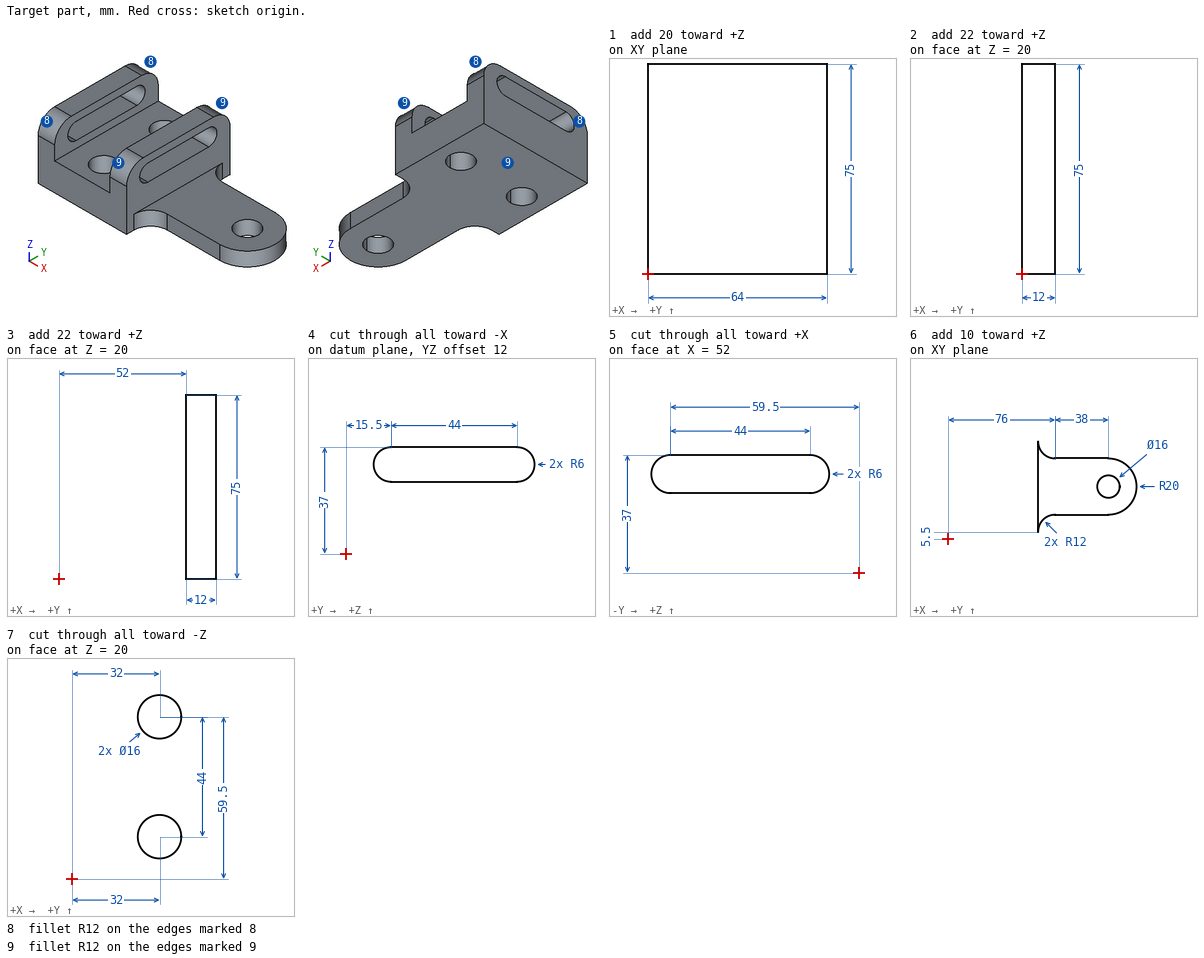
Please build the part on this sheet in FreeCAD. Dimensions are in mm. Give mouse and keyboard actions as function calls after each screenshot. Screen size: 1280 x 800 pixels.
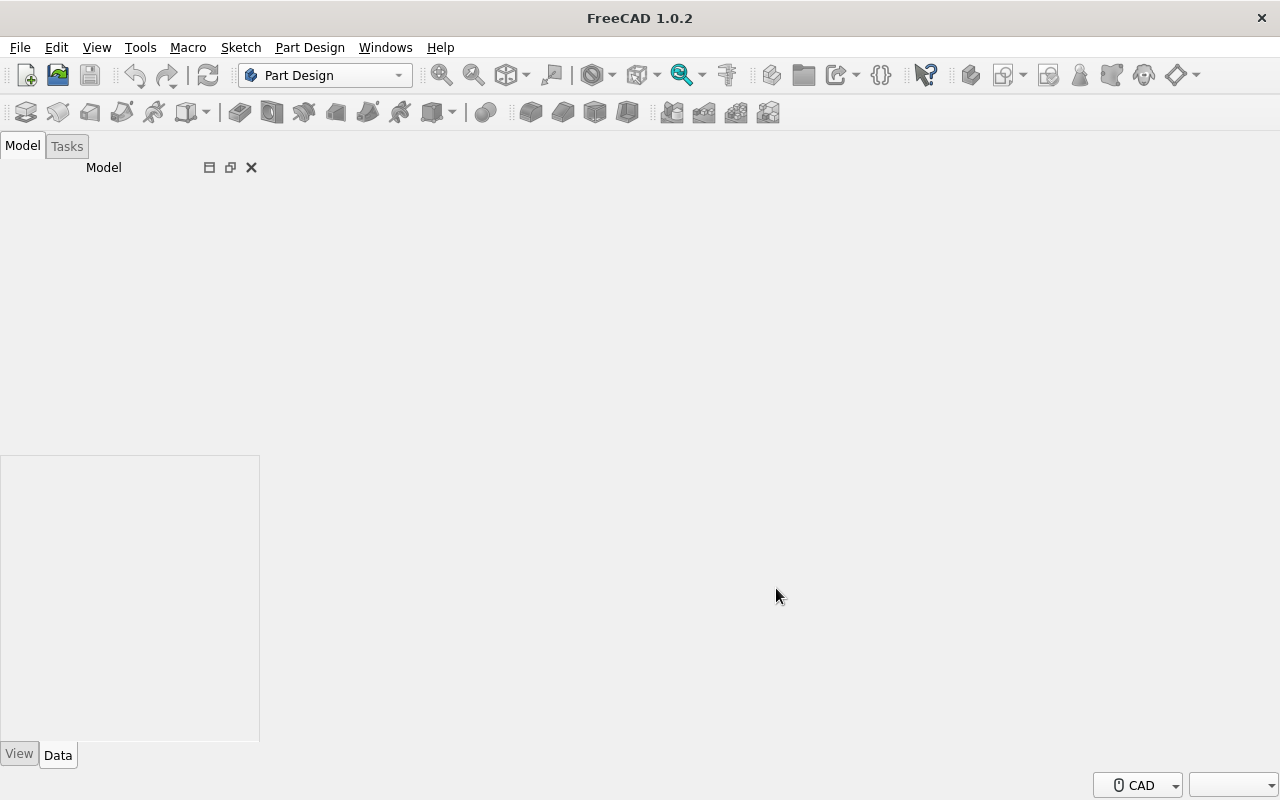
click(26, 76)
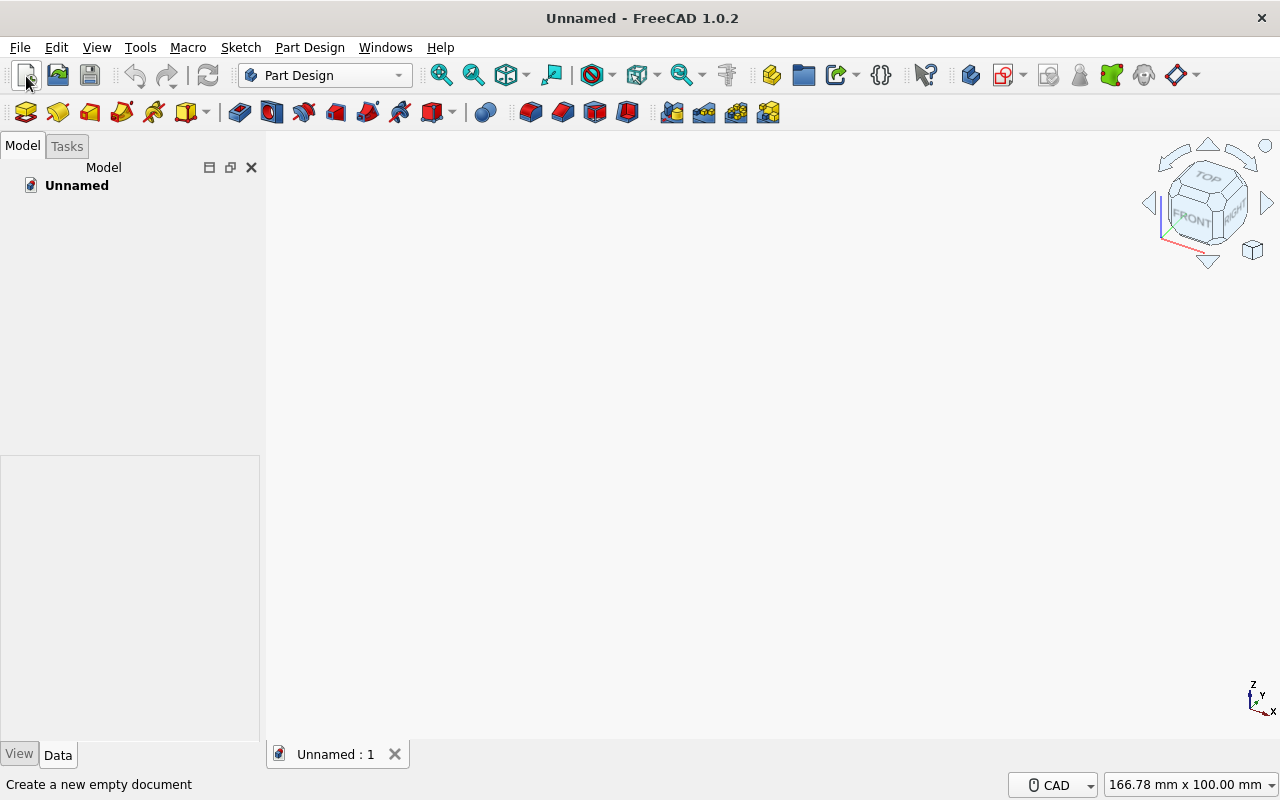
click(1004, 76)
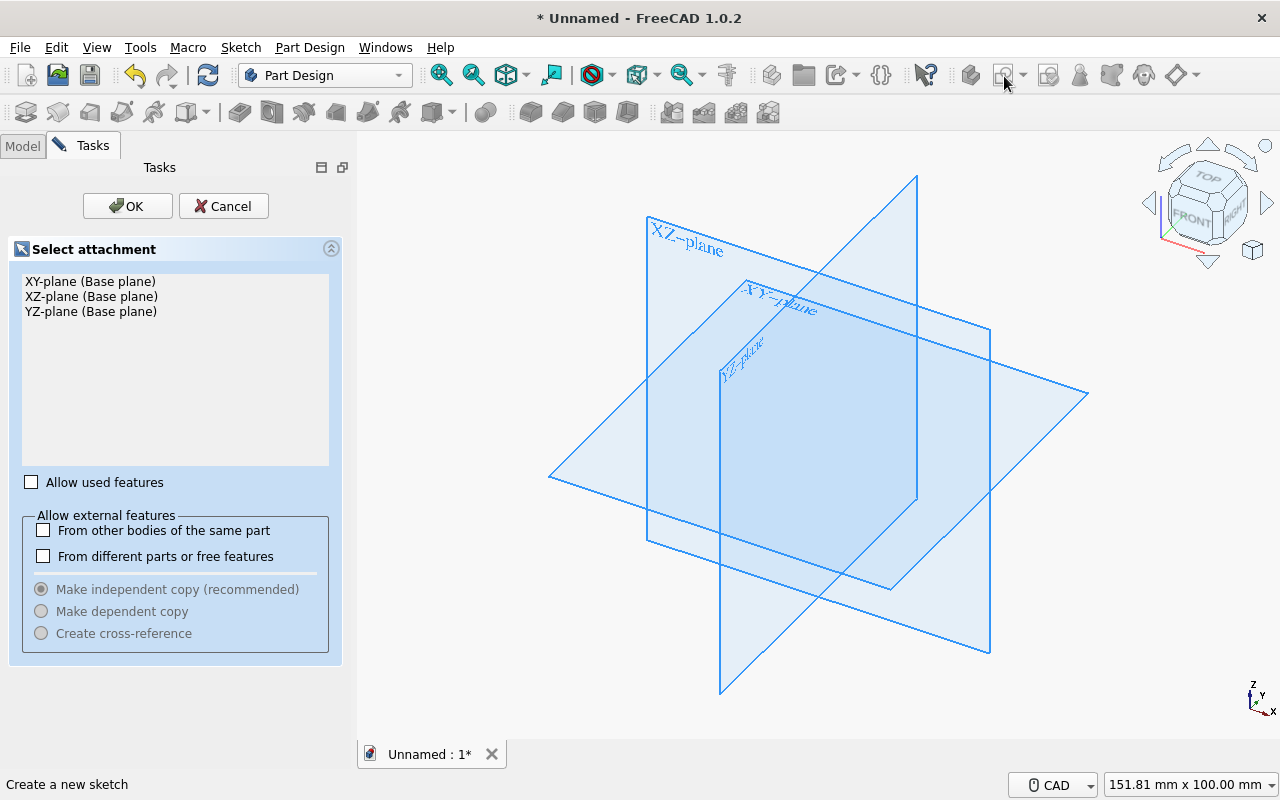
click(82, 282)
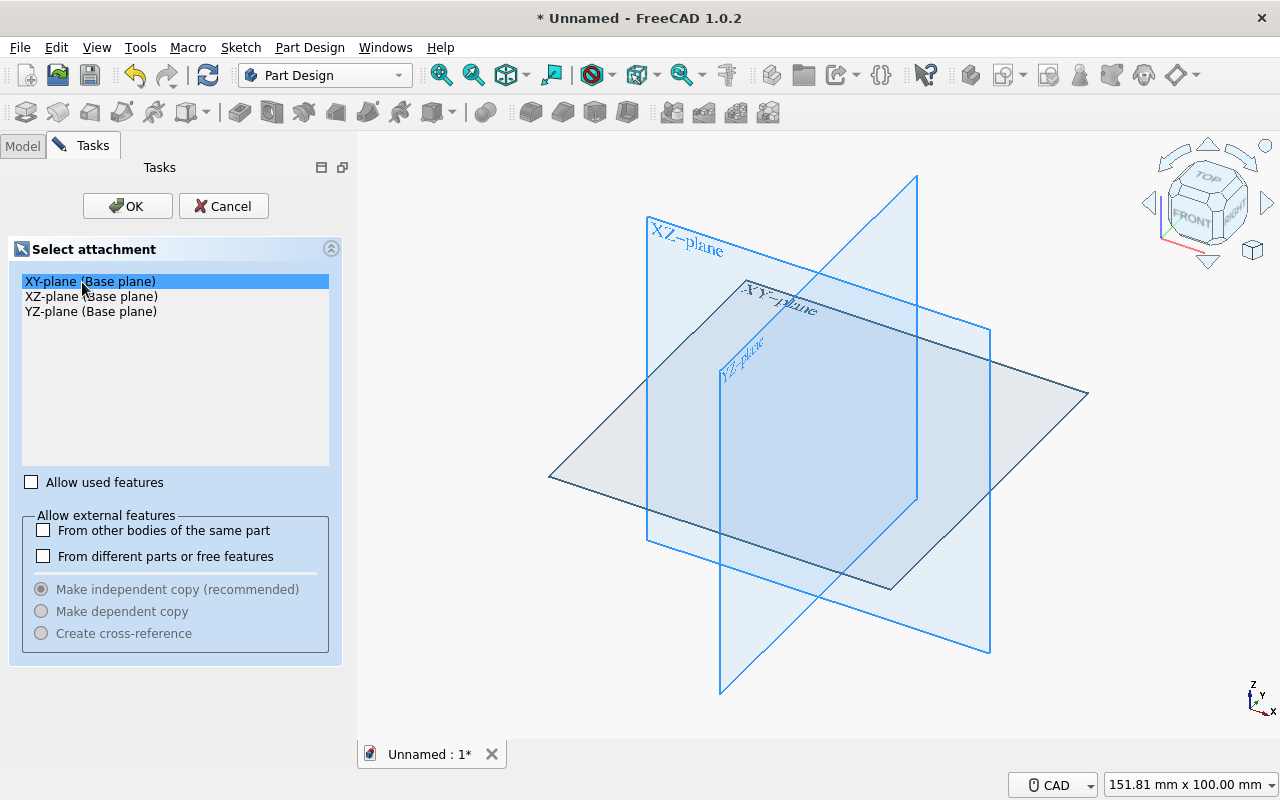
click(128, 206)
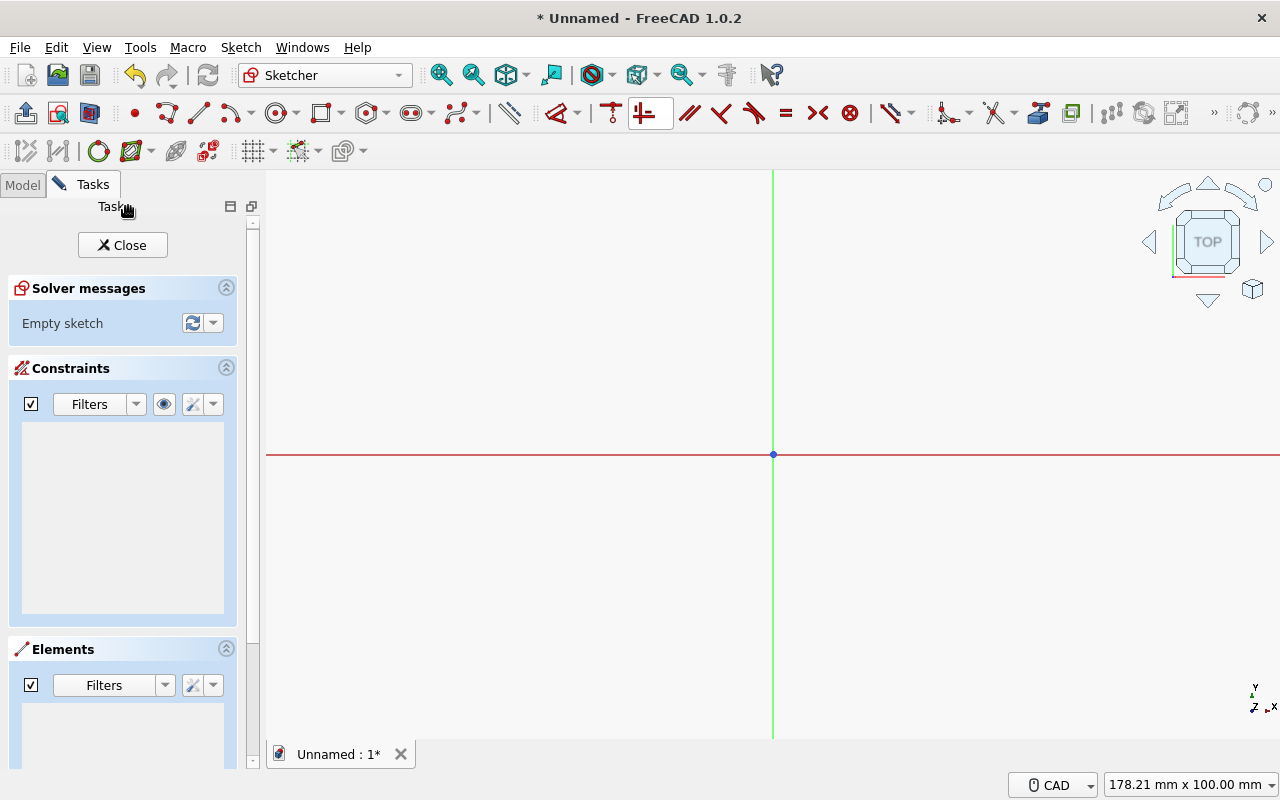
scroll(294, 711, down, 2)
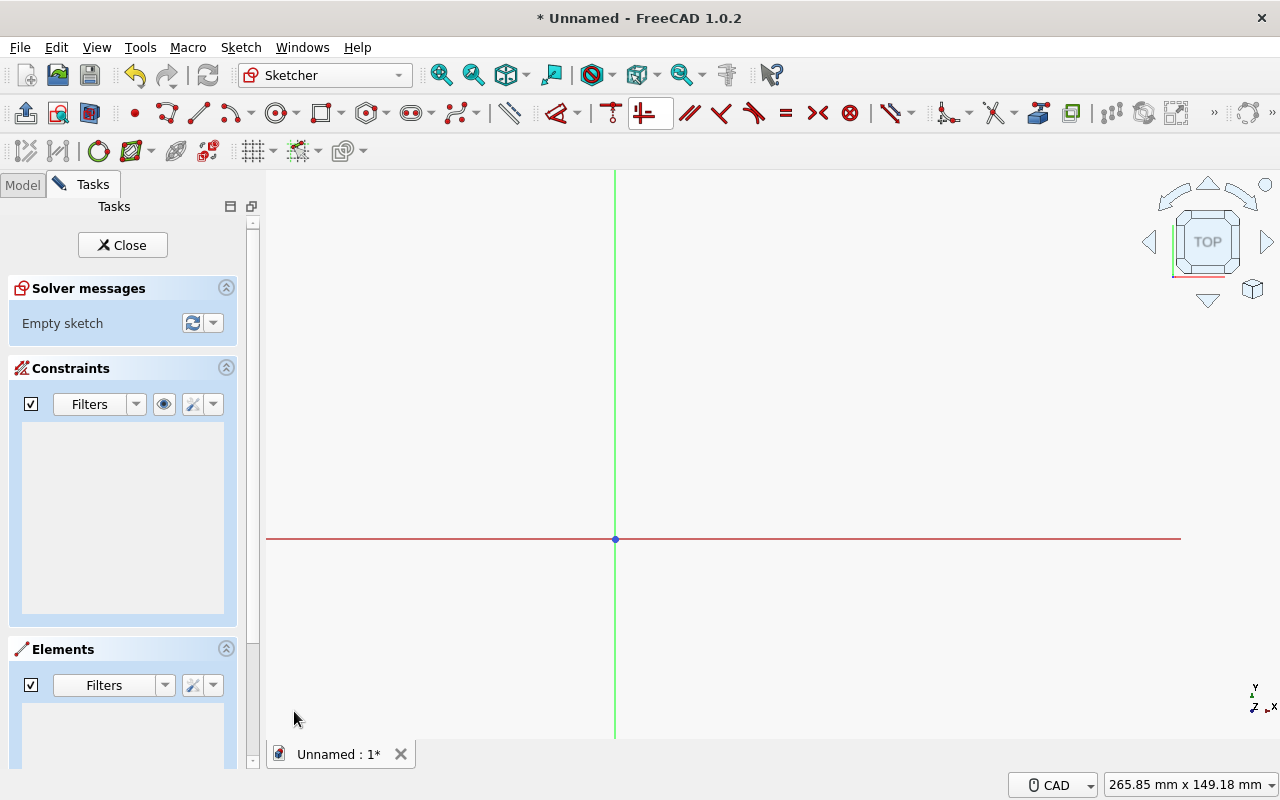
click(322, 114)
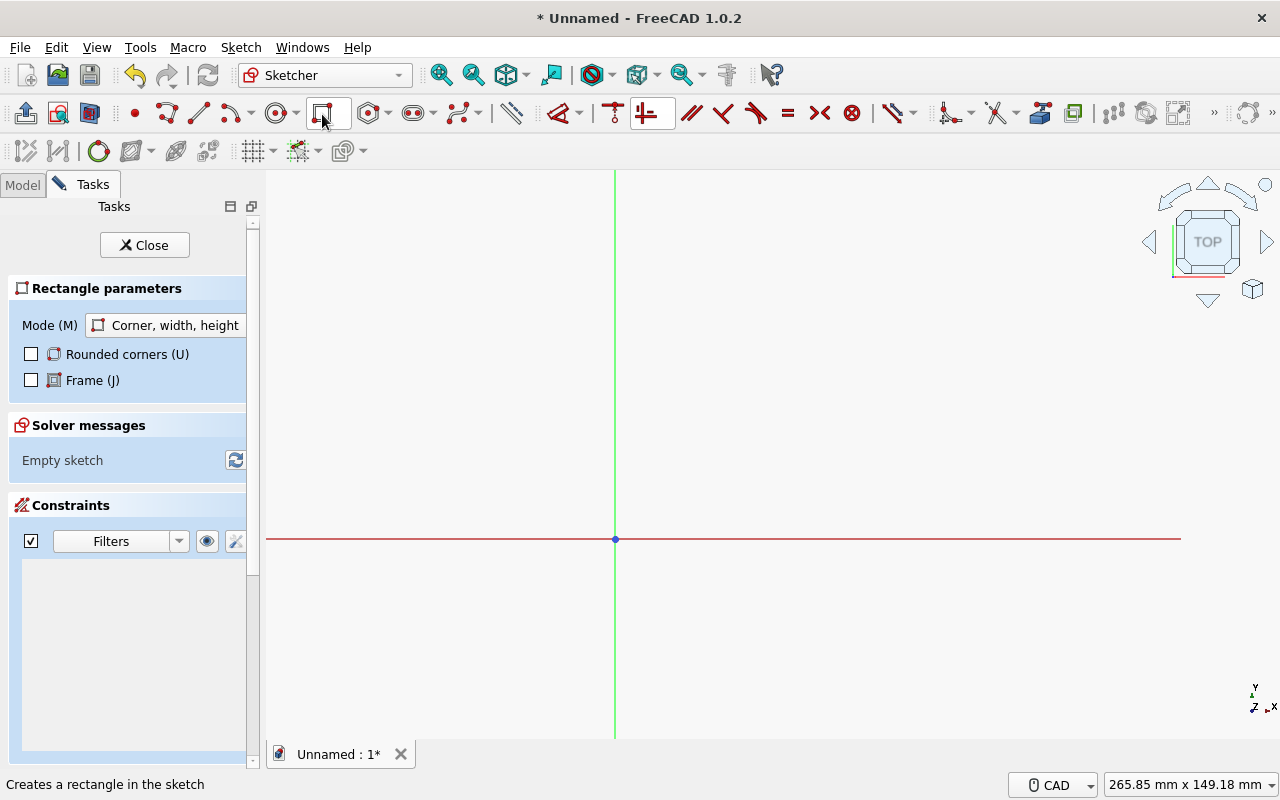
click(615, 539)
click(859, 253)
key(Escape)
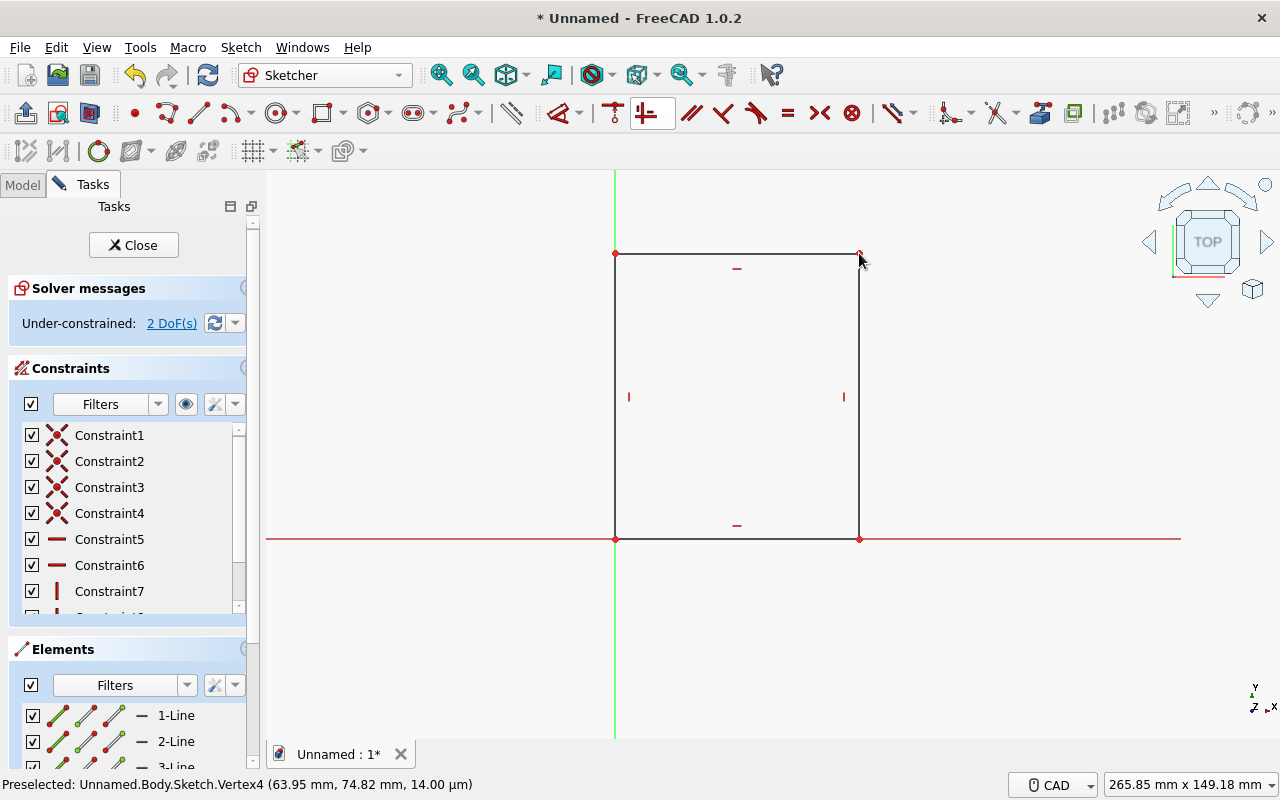
click(558, 114)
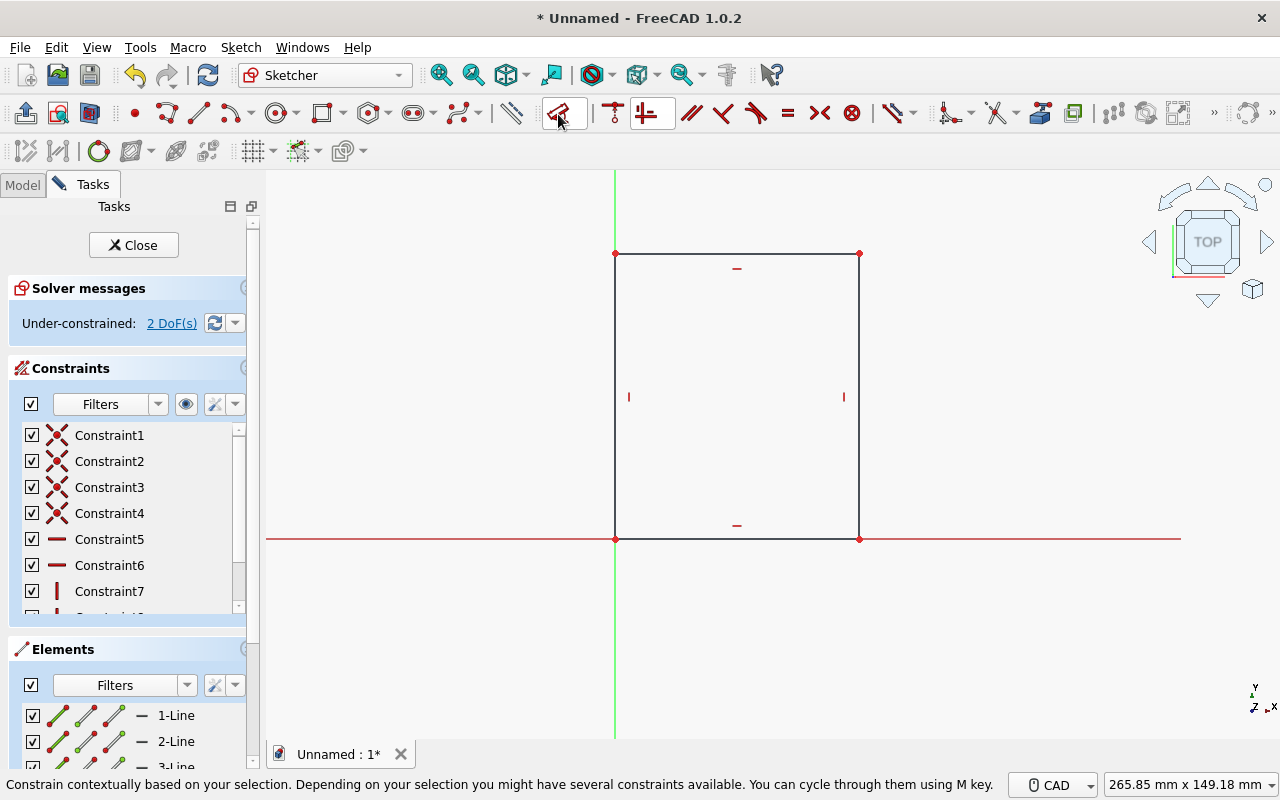
click(688, 539)
click(737, 573)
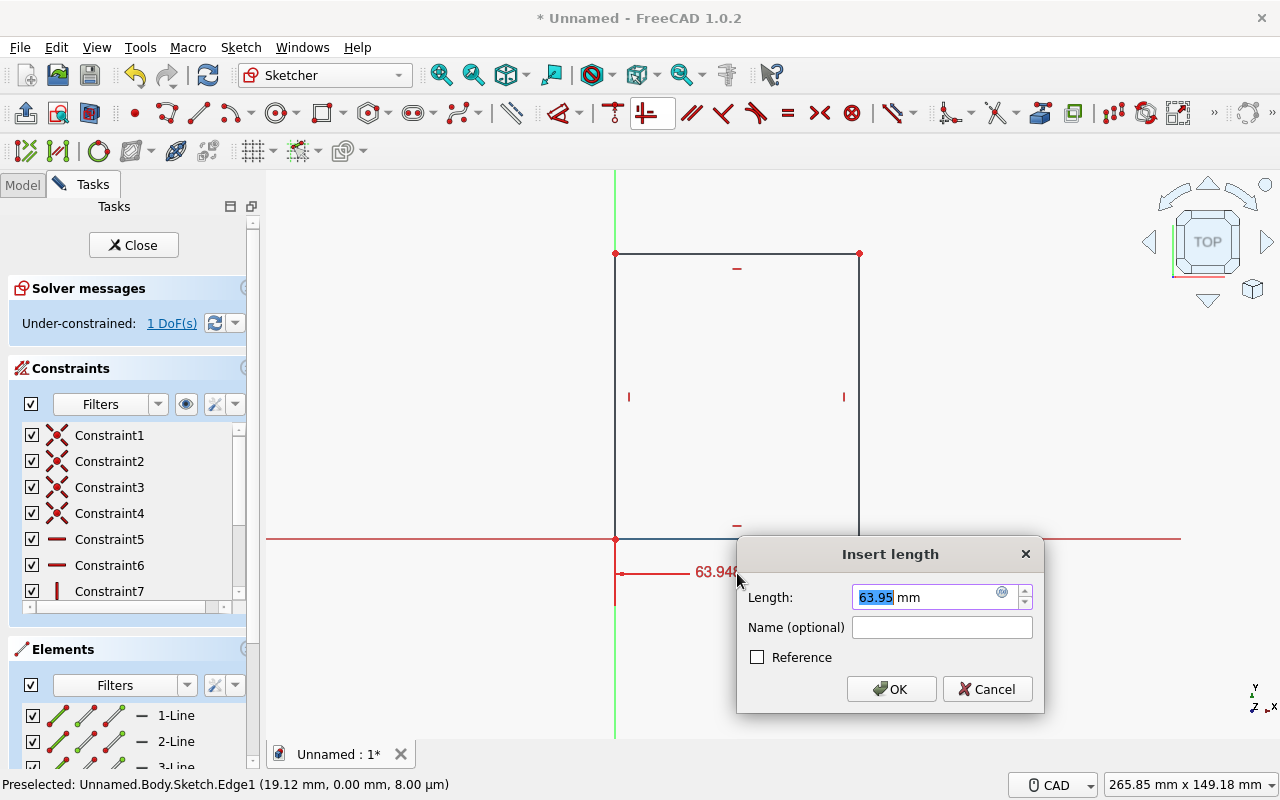
text(64)
key(Return)